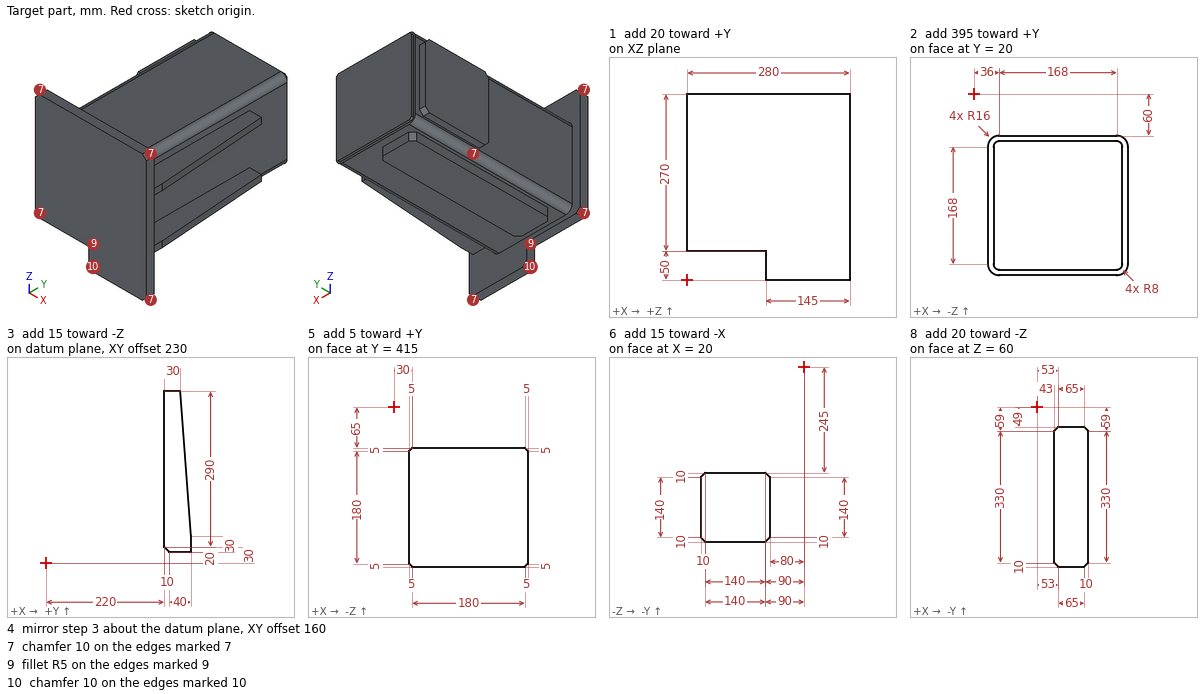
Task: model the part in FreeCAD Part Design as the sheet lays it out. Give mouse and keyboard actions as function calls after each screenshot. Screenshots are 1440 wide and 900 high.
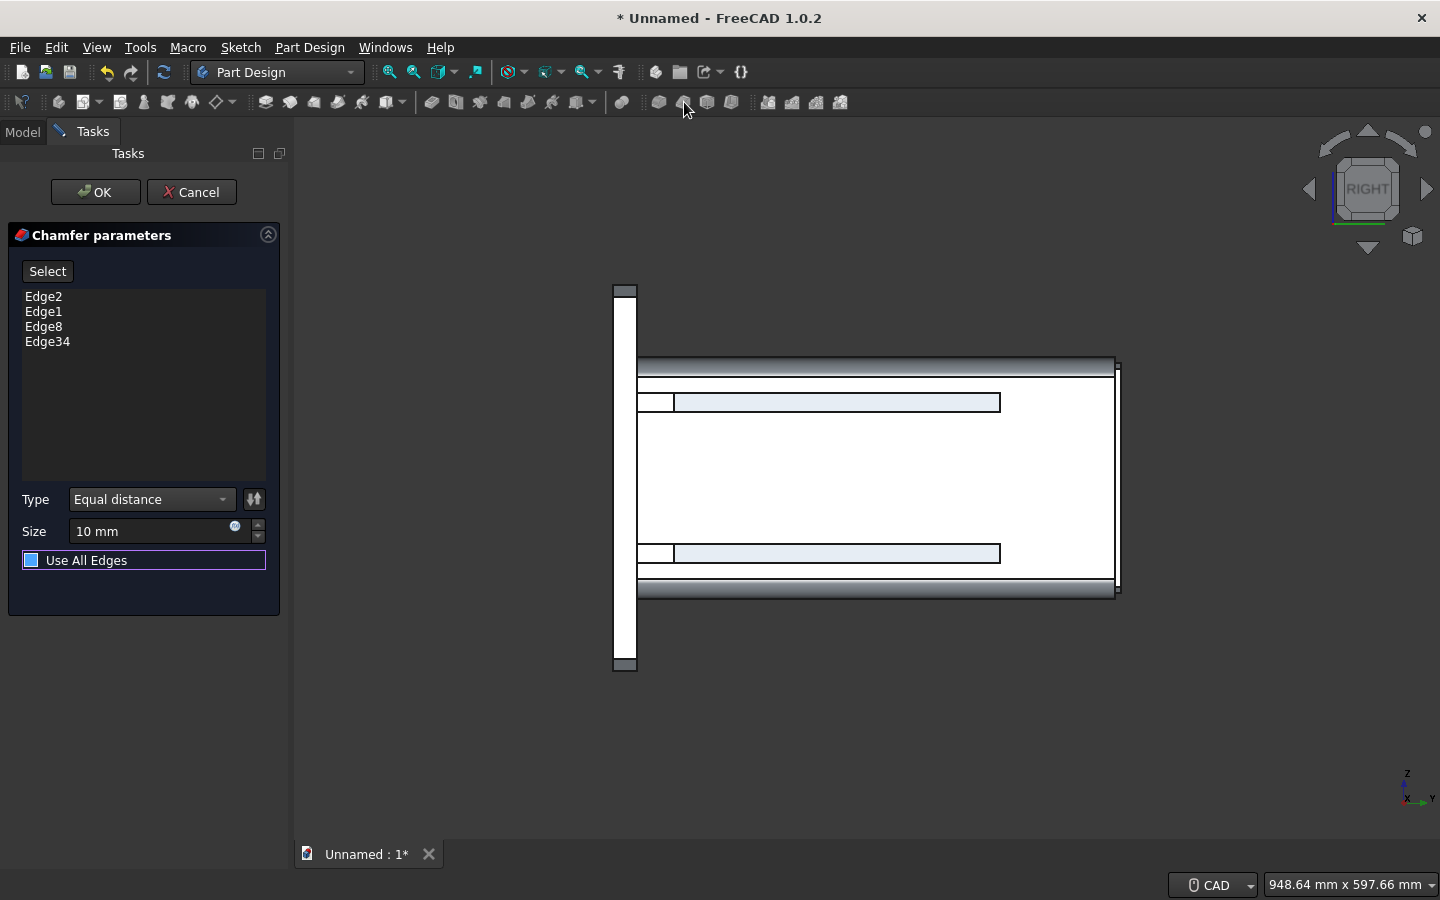
click(96, 192)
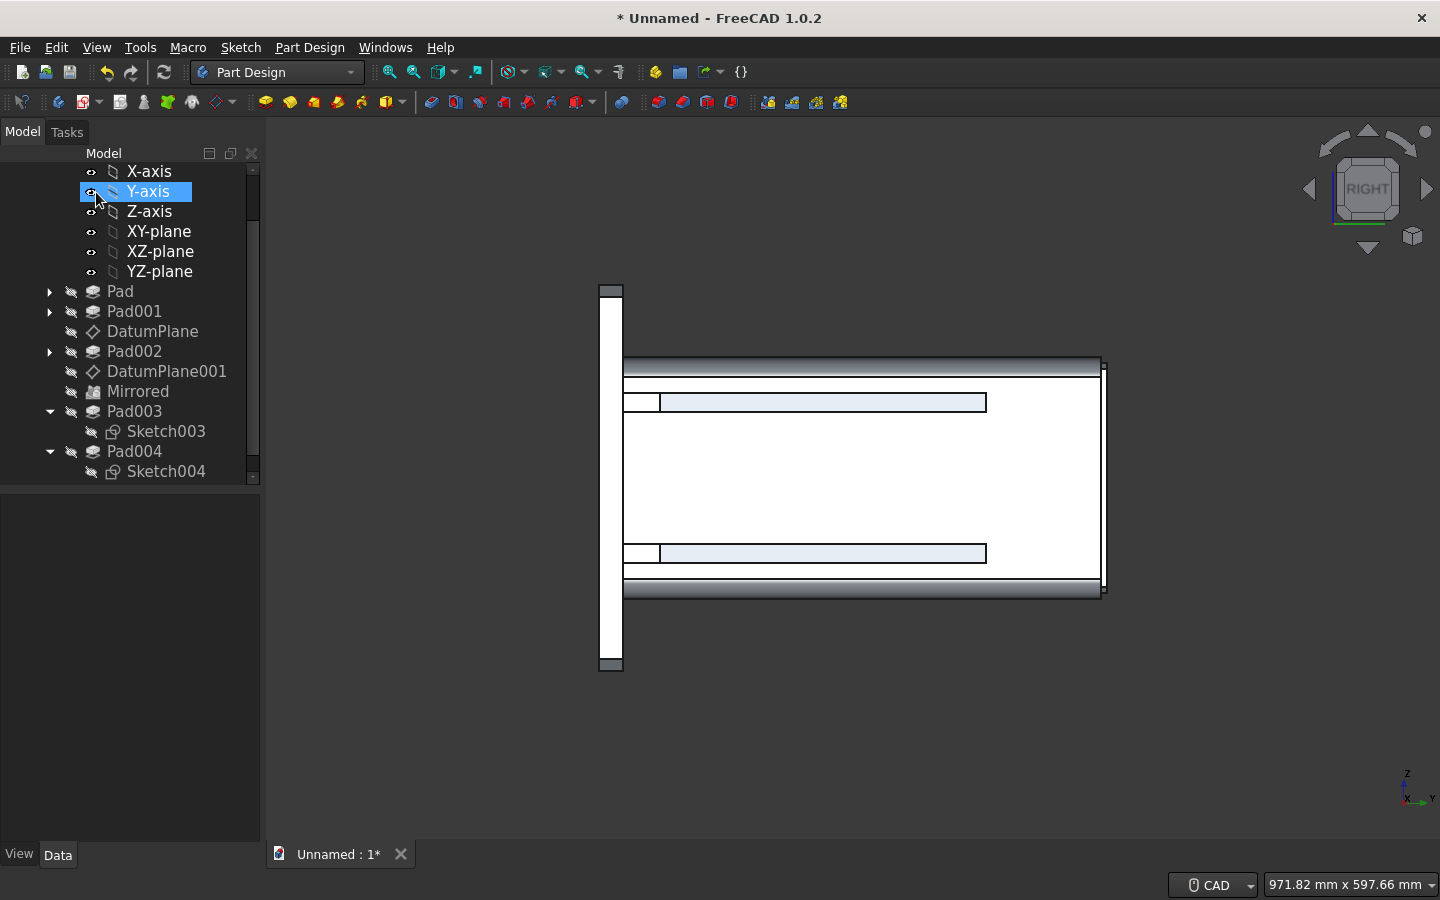
key(5)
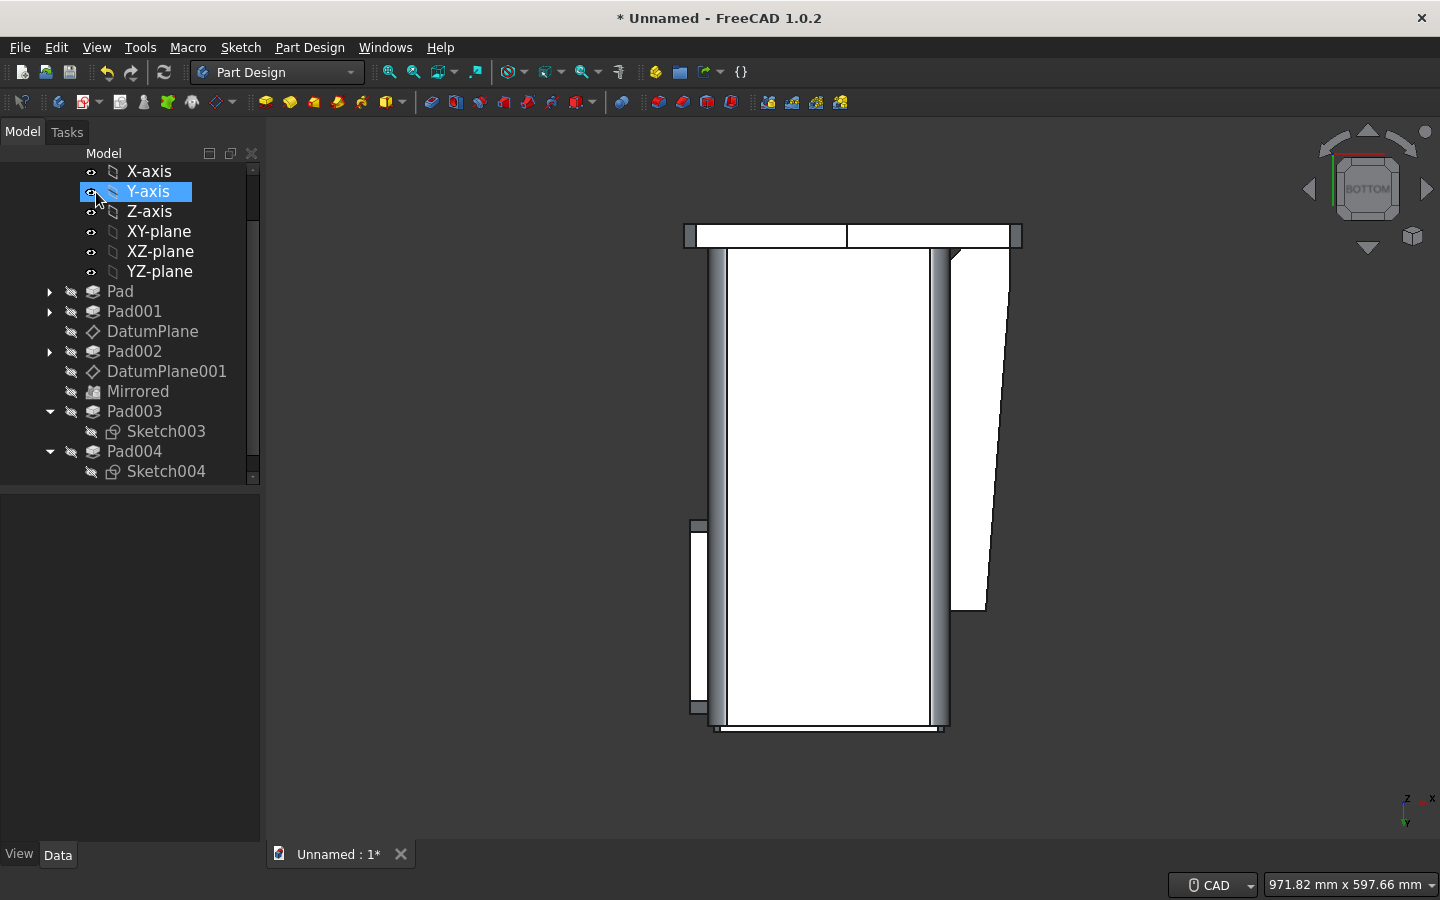
click(829, 622)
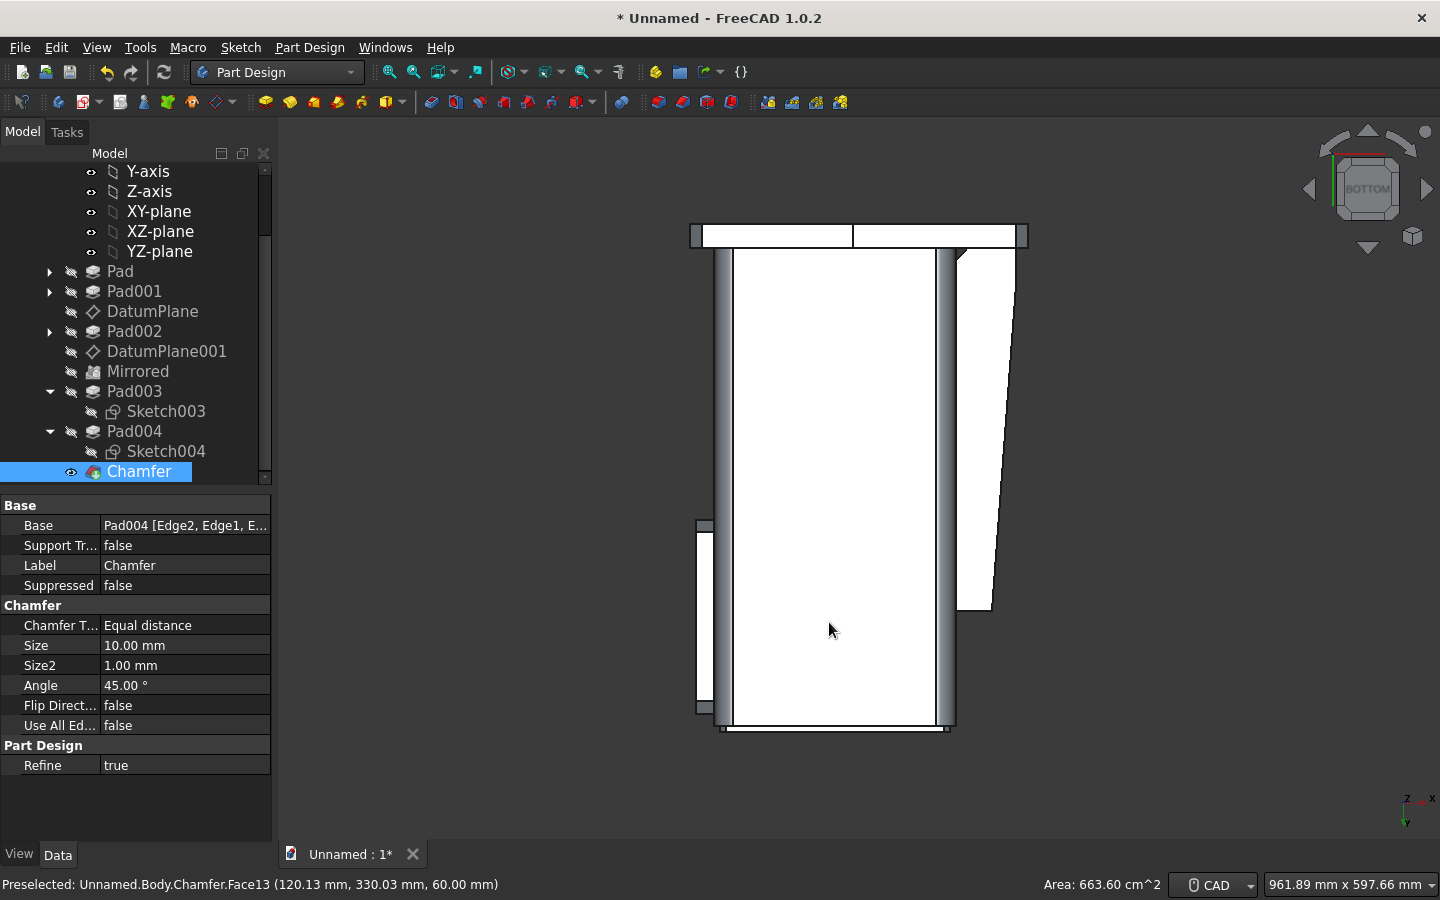
click(84, 102)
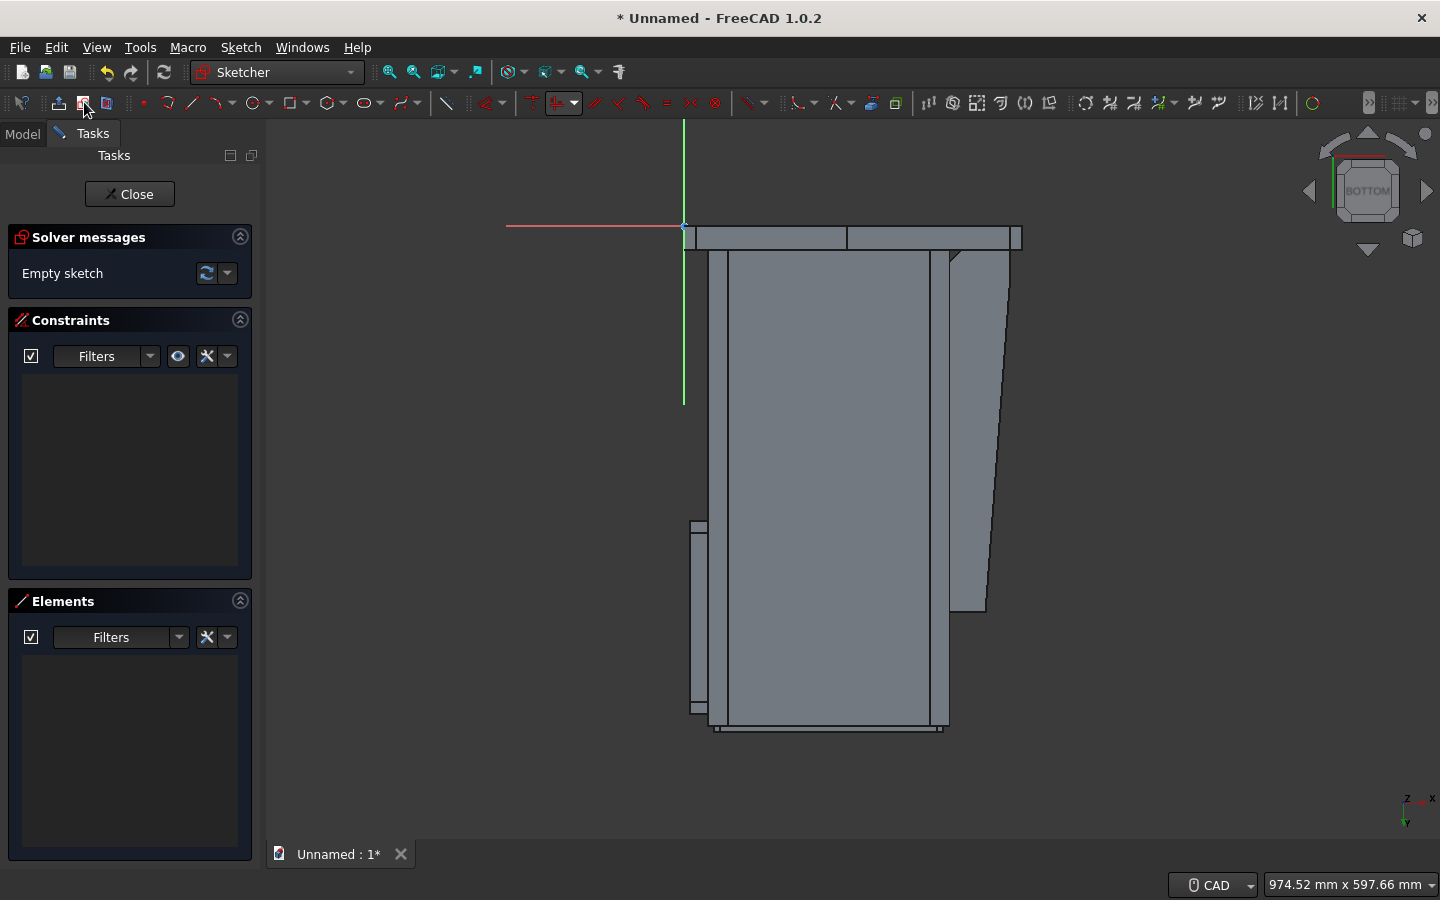
click(168, 104)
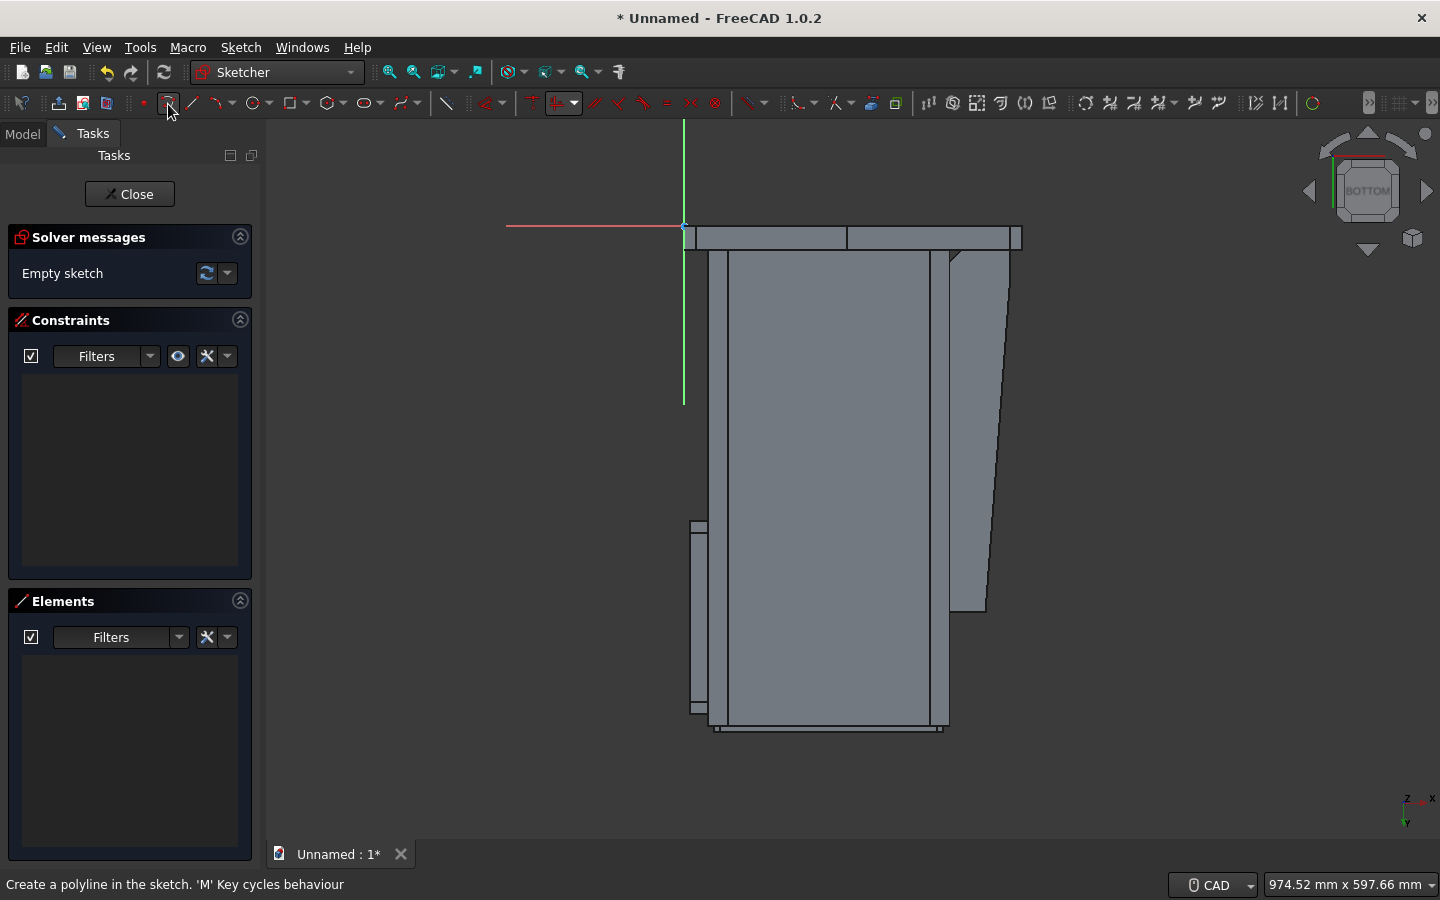
click(748, 285)
click(736, 297)
click(736, 695)
click(748, 707)
click(826, 707)
click(839, 695)
click(839, 297)
click(826, 285)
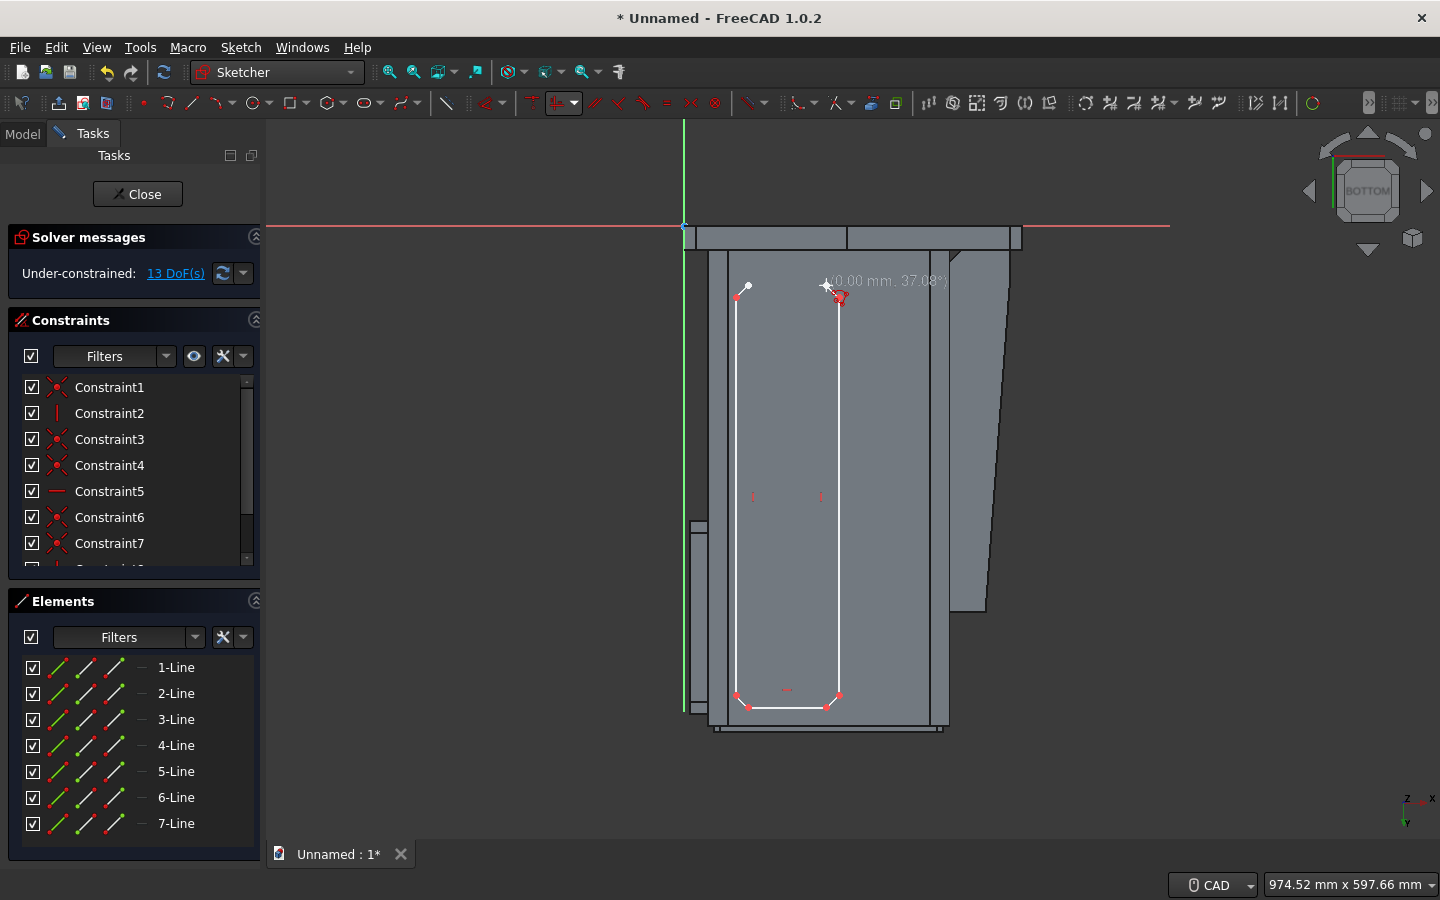
scroll(748, 285, up, 4)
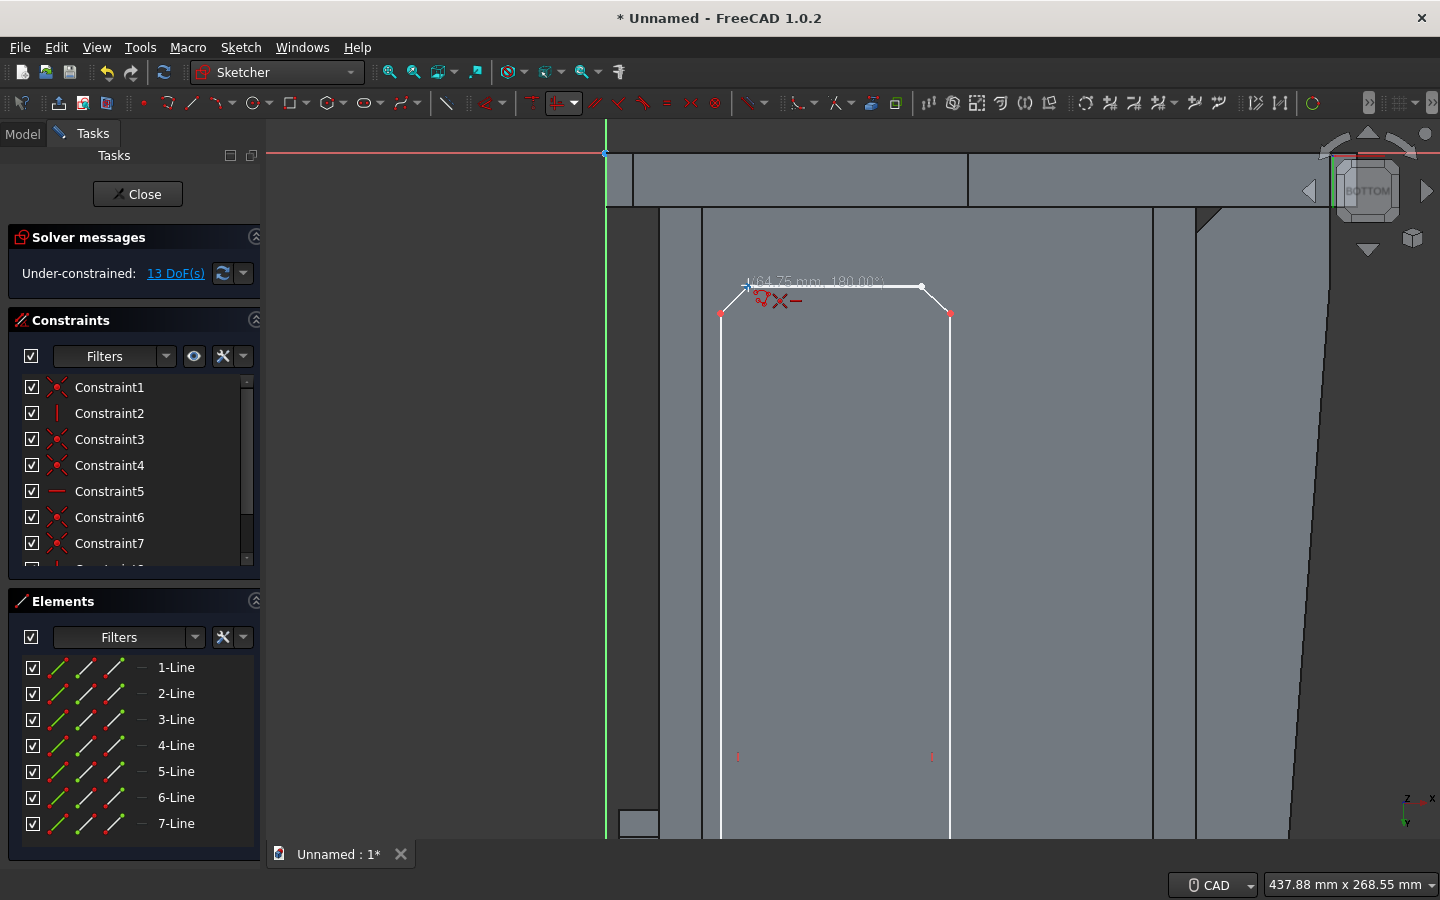
click(747, 287)
key(Escape)
key(Escape)